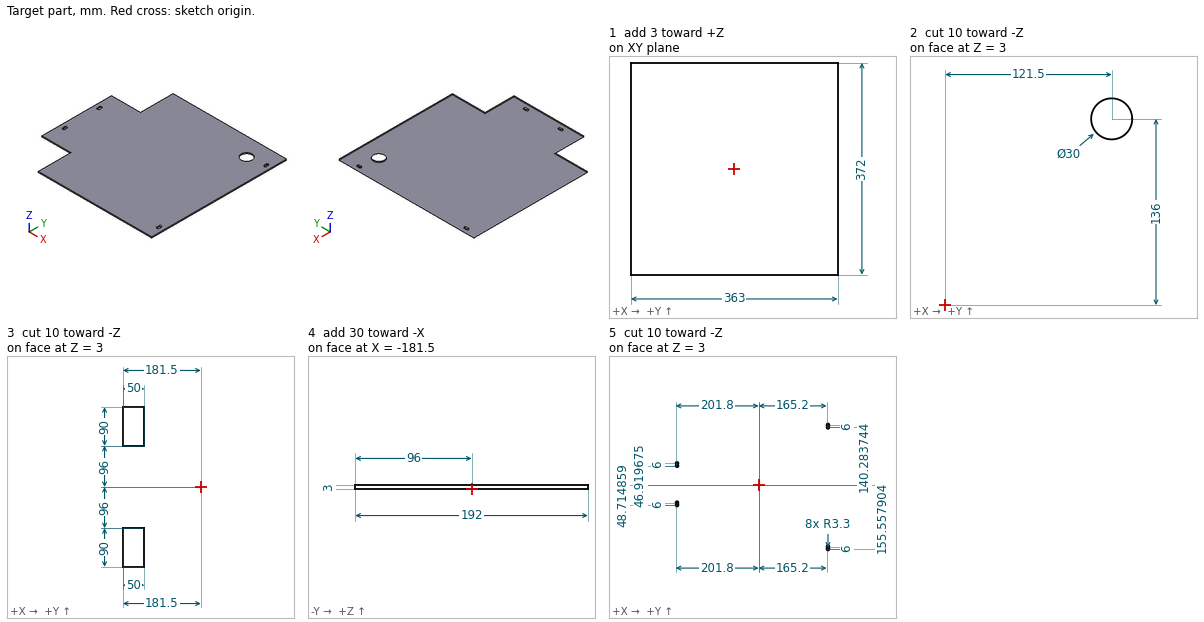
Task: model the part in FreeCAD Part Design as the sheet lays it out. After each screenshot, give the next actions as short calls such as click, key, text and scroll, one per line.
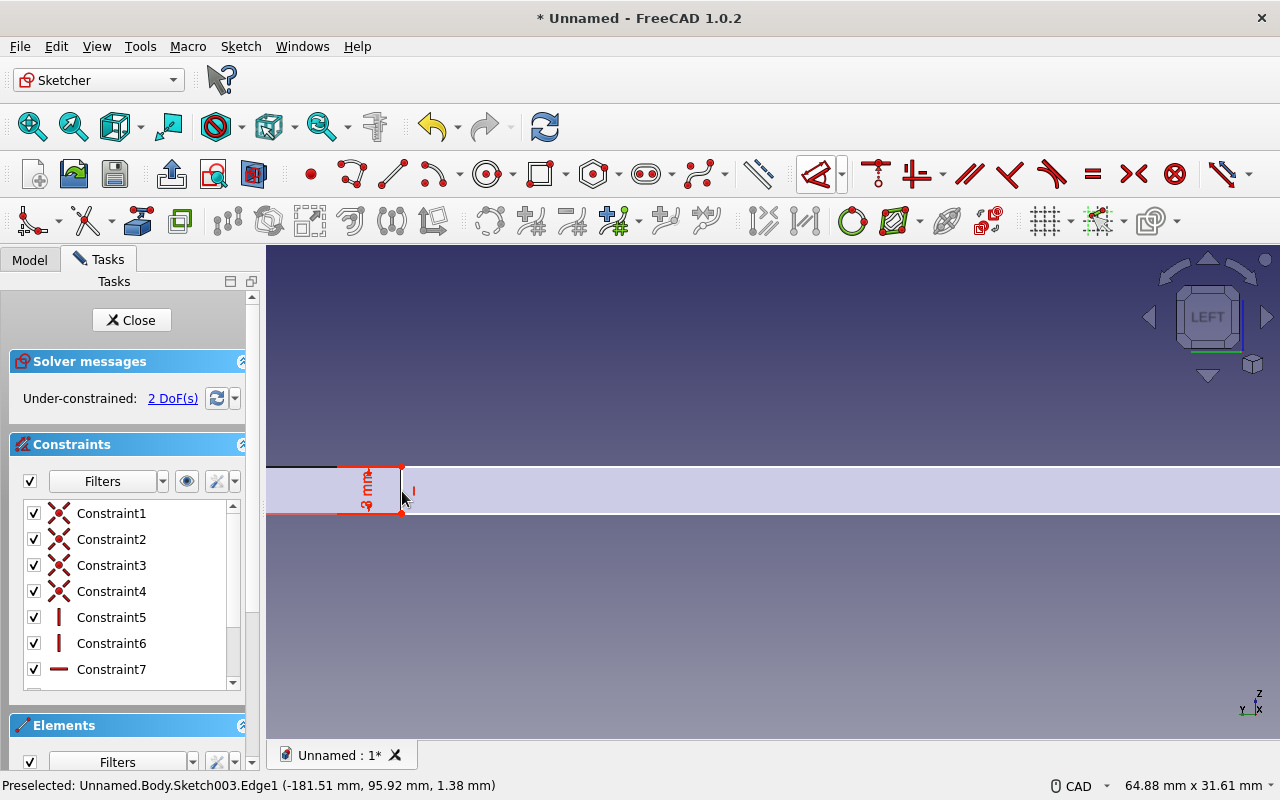
scroll(402, 492, down, 8)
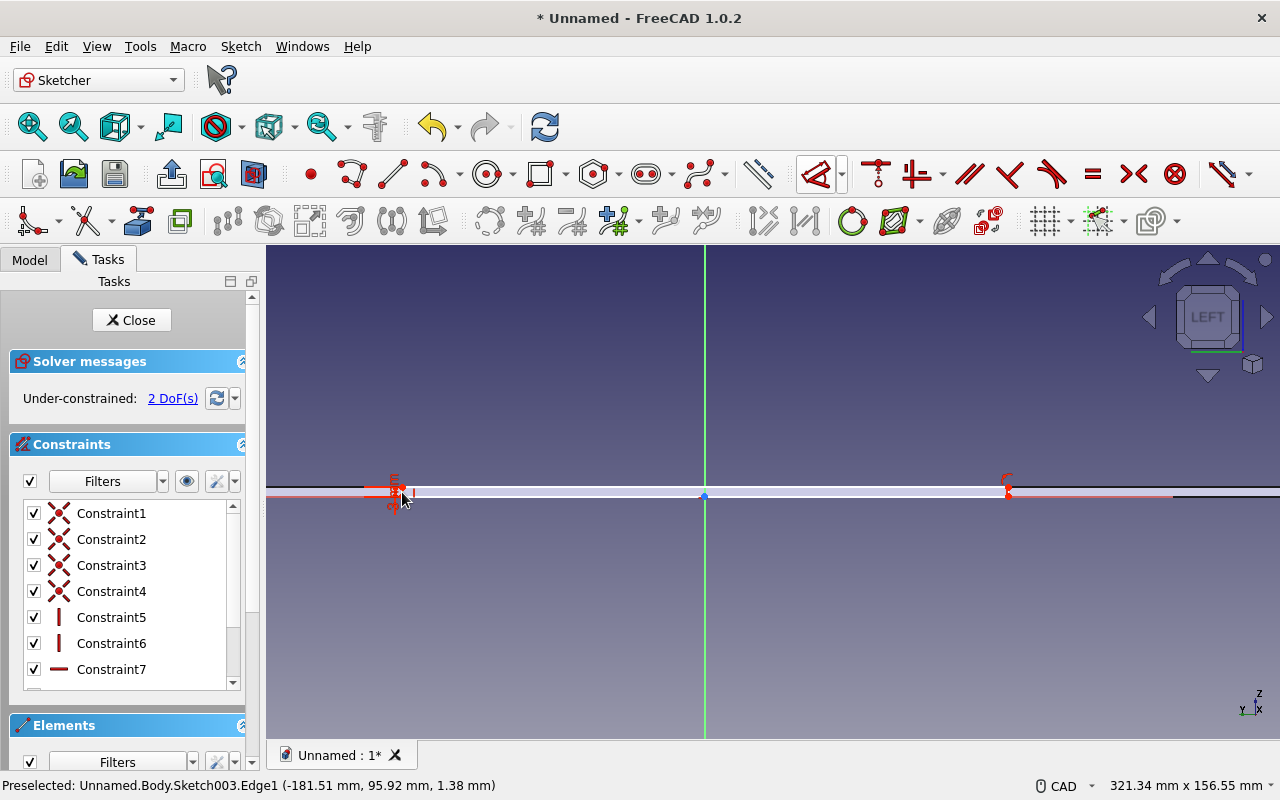
scroll(523, 497, up, 2)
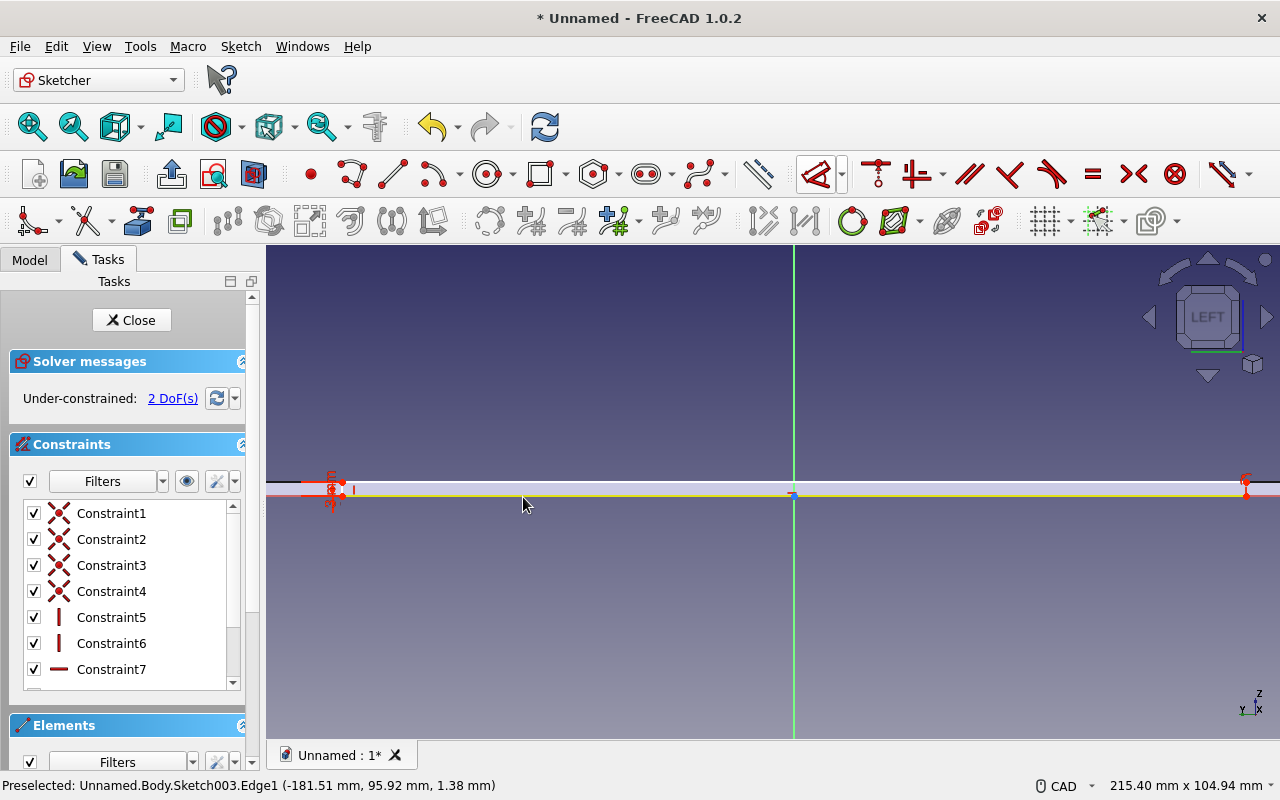
click(523, 496)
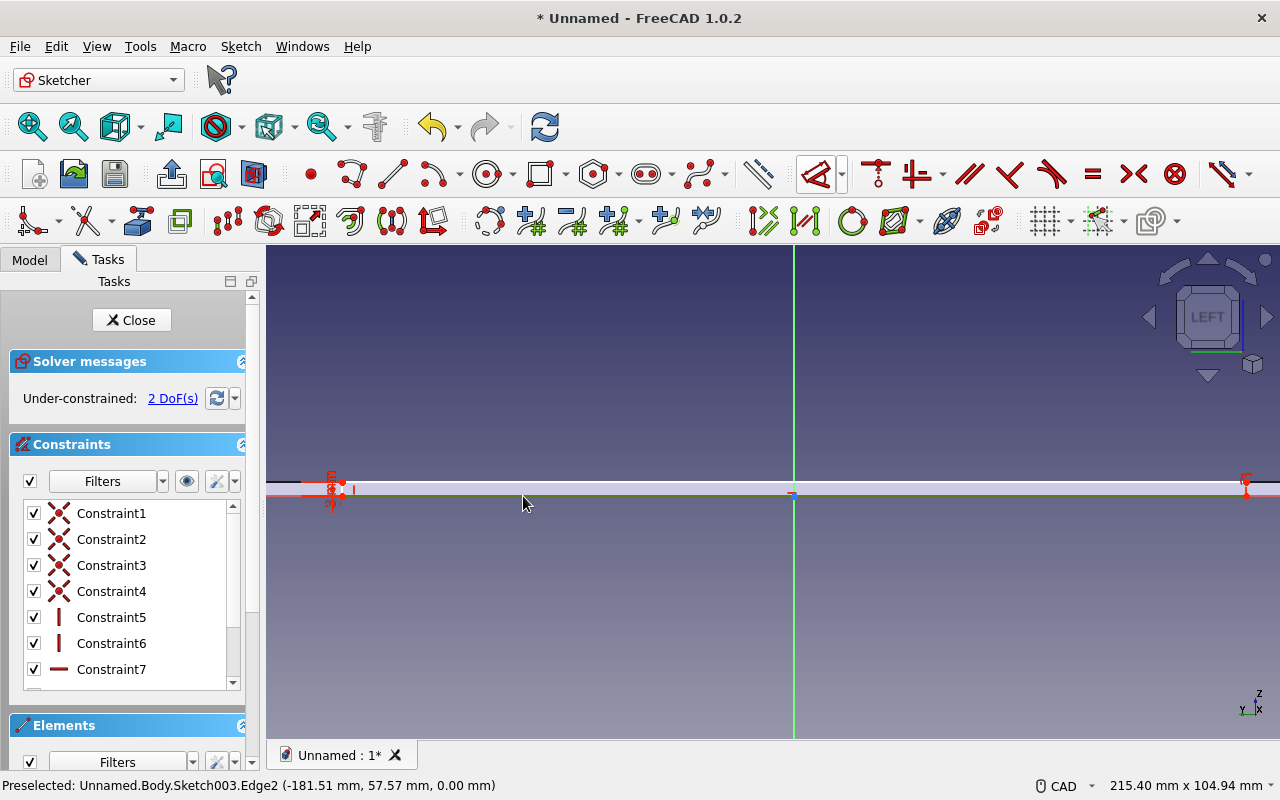
key(l)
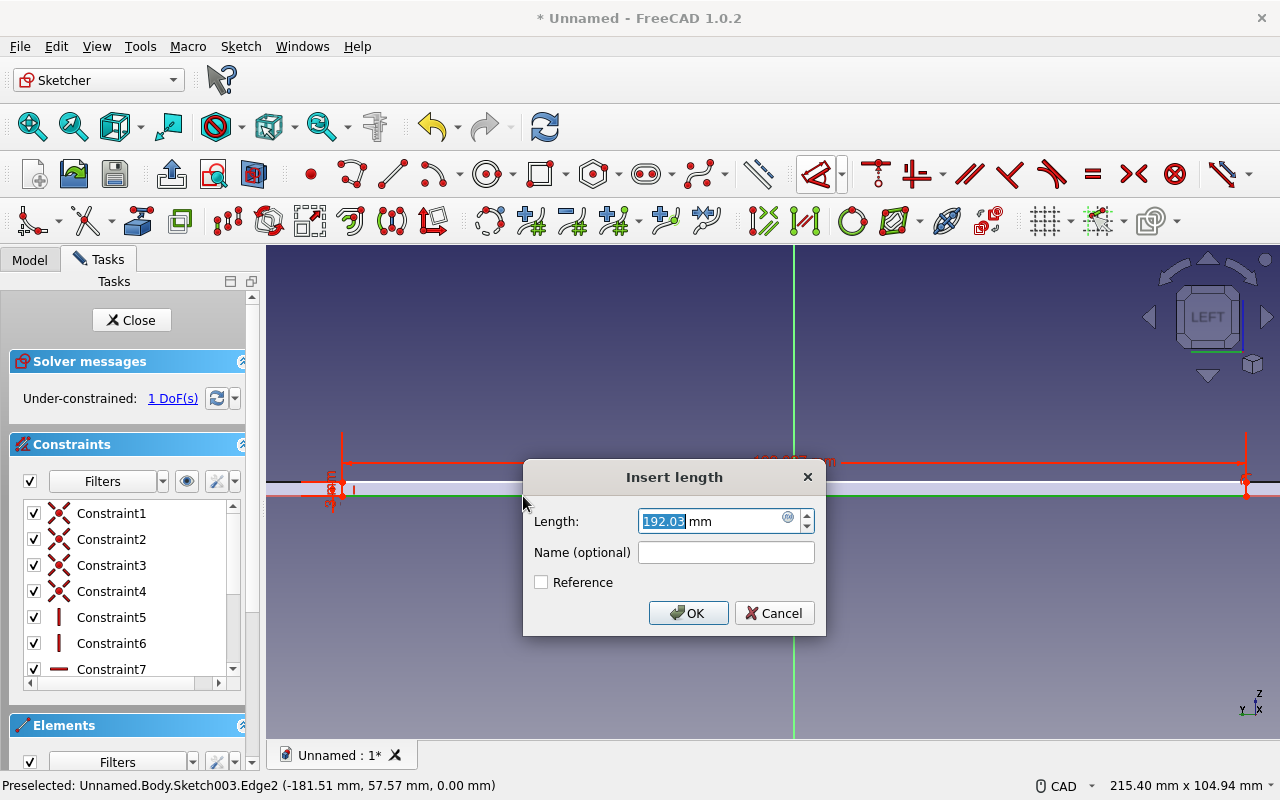
text(192)
key(Return)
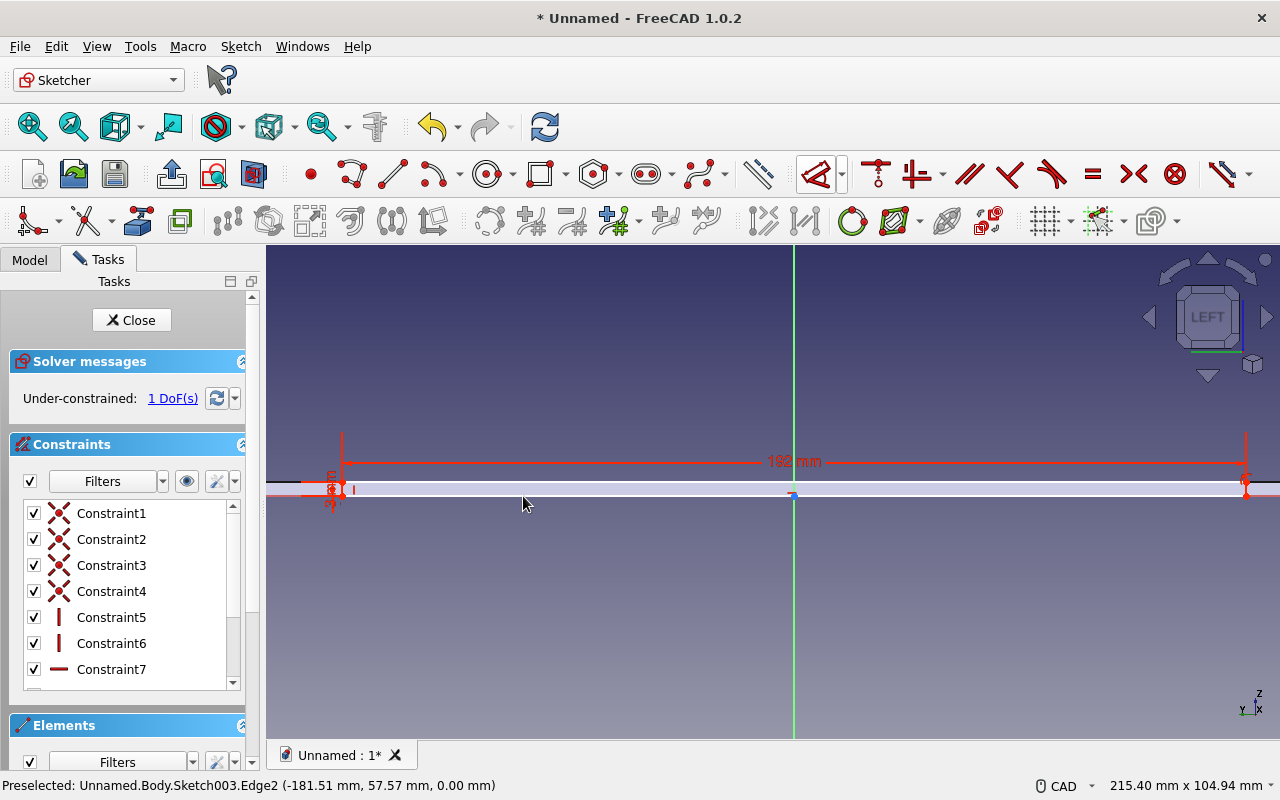
click(342, 482)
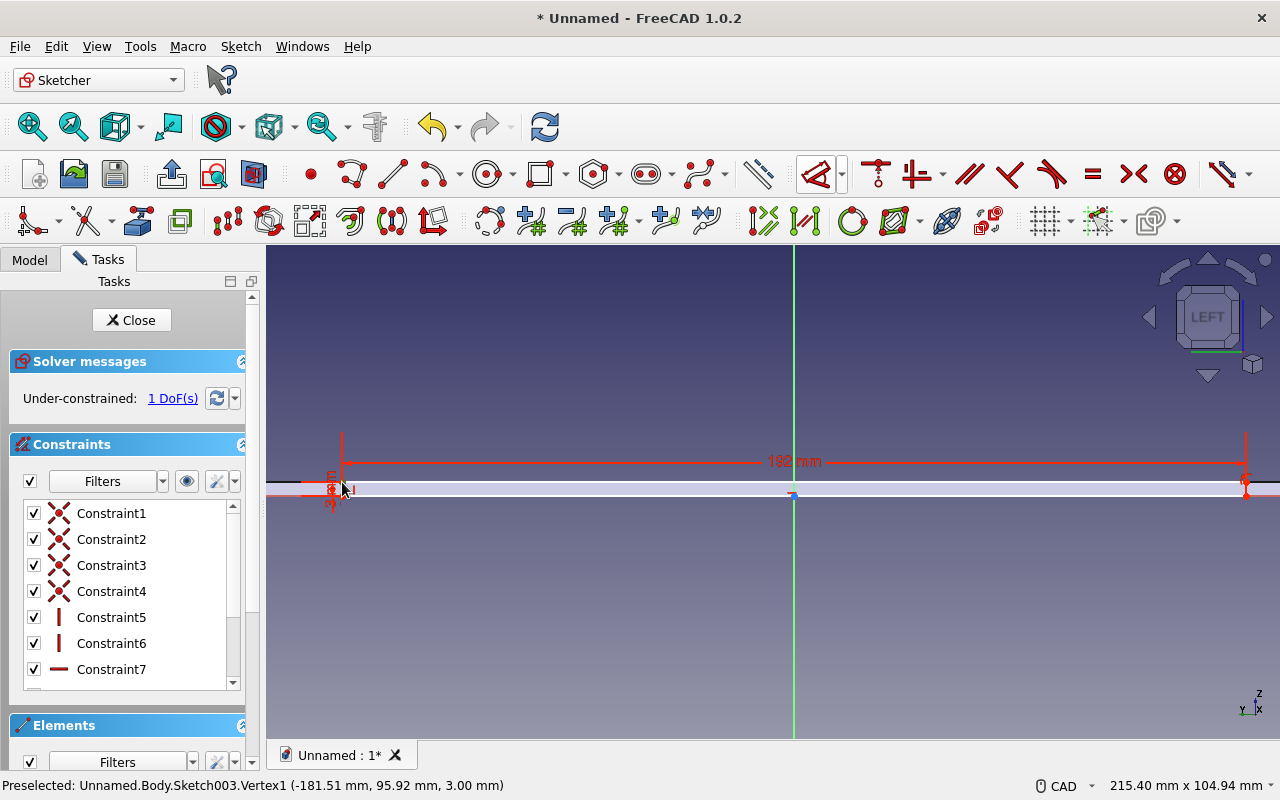
key(l)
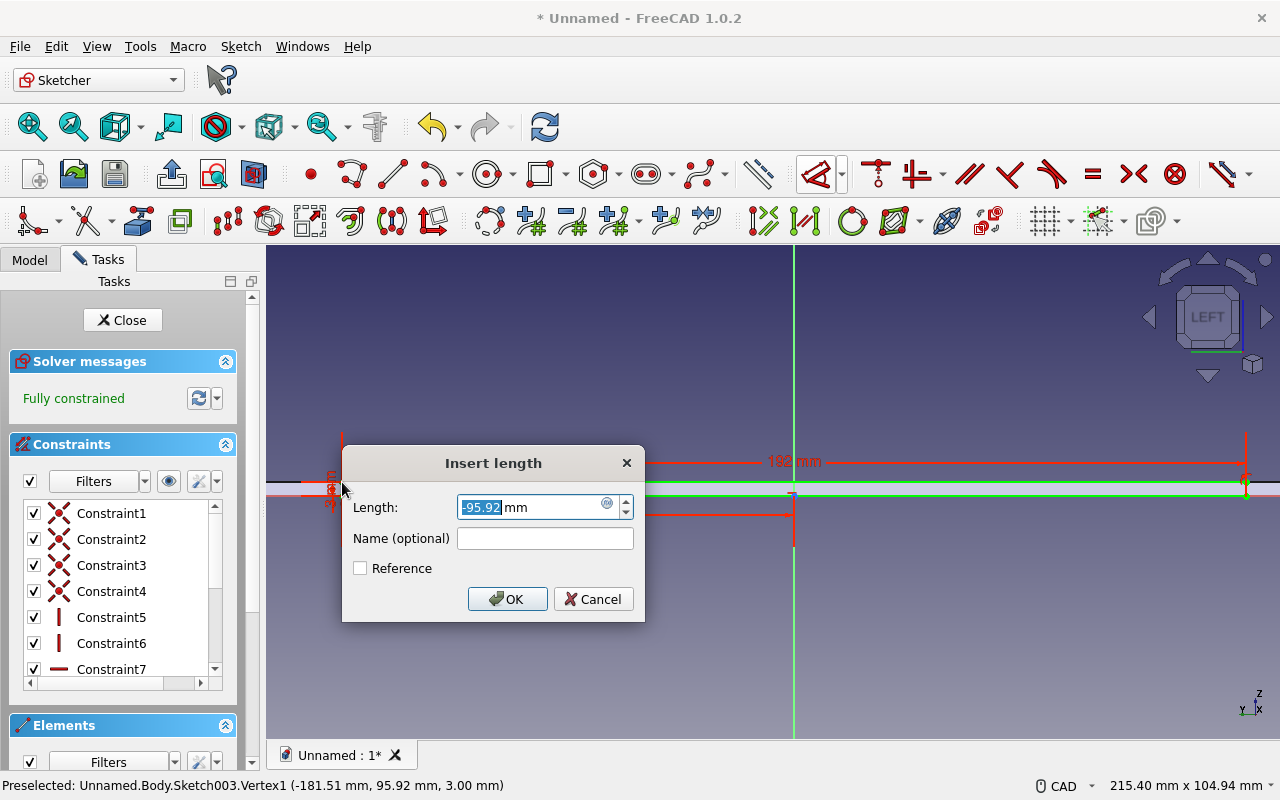
text(-96)
key(Return)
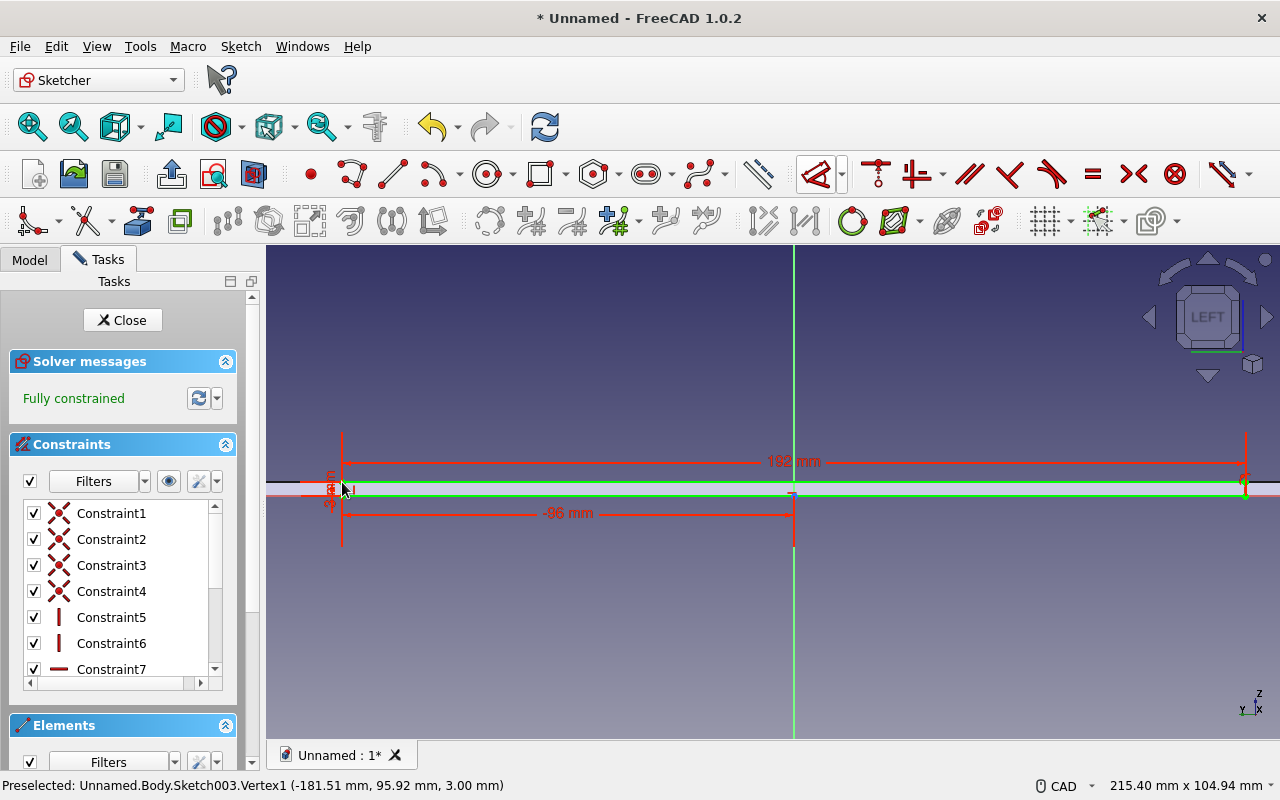
click(123, 320)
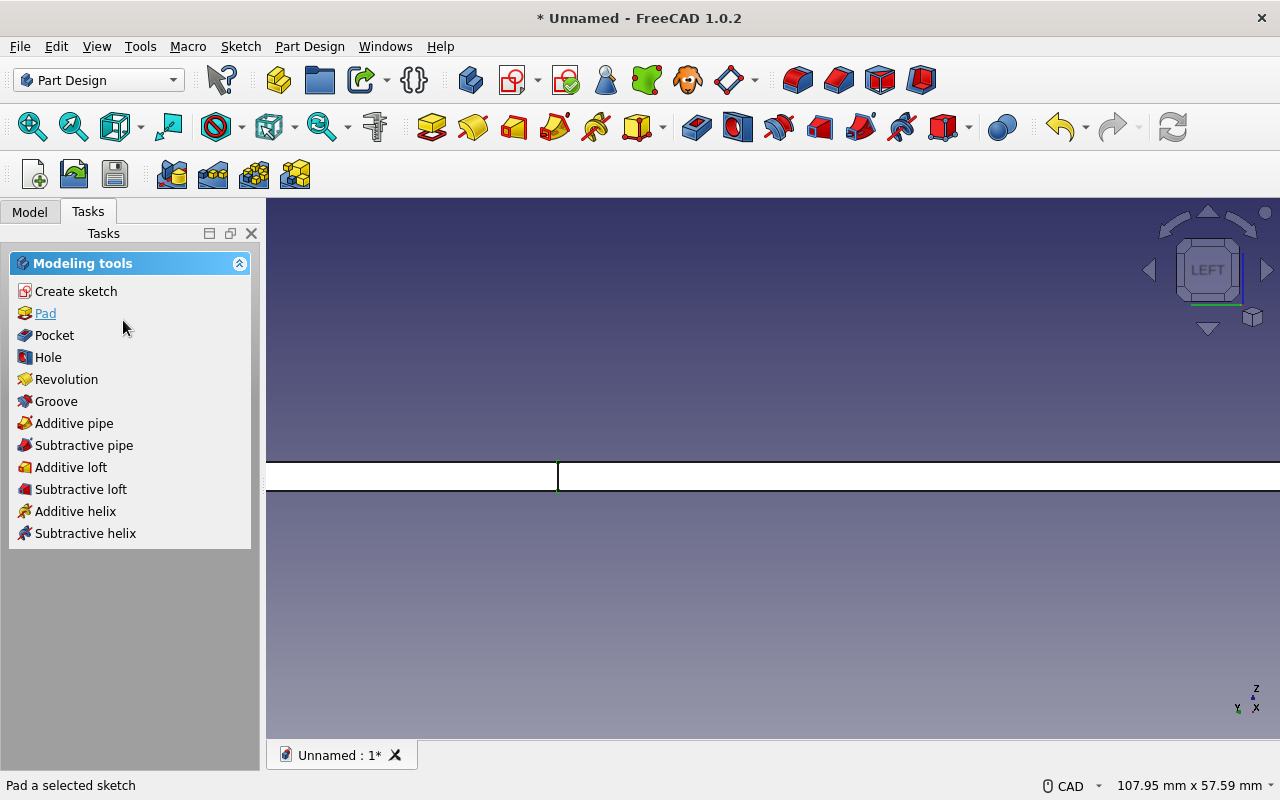
click(432, 128)